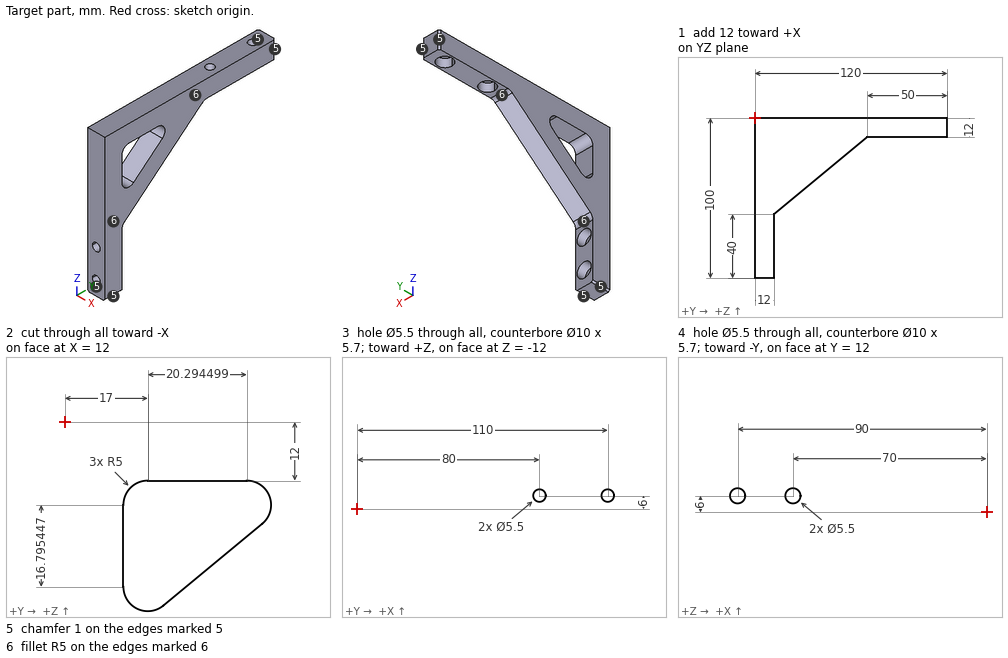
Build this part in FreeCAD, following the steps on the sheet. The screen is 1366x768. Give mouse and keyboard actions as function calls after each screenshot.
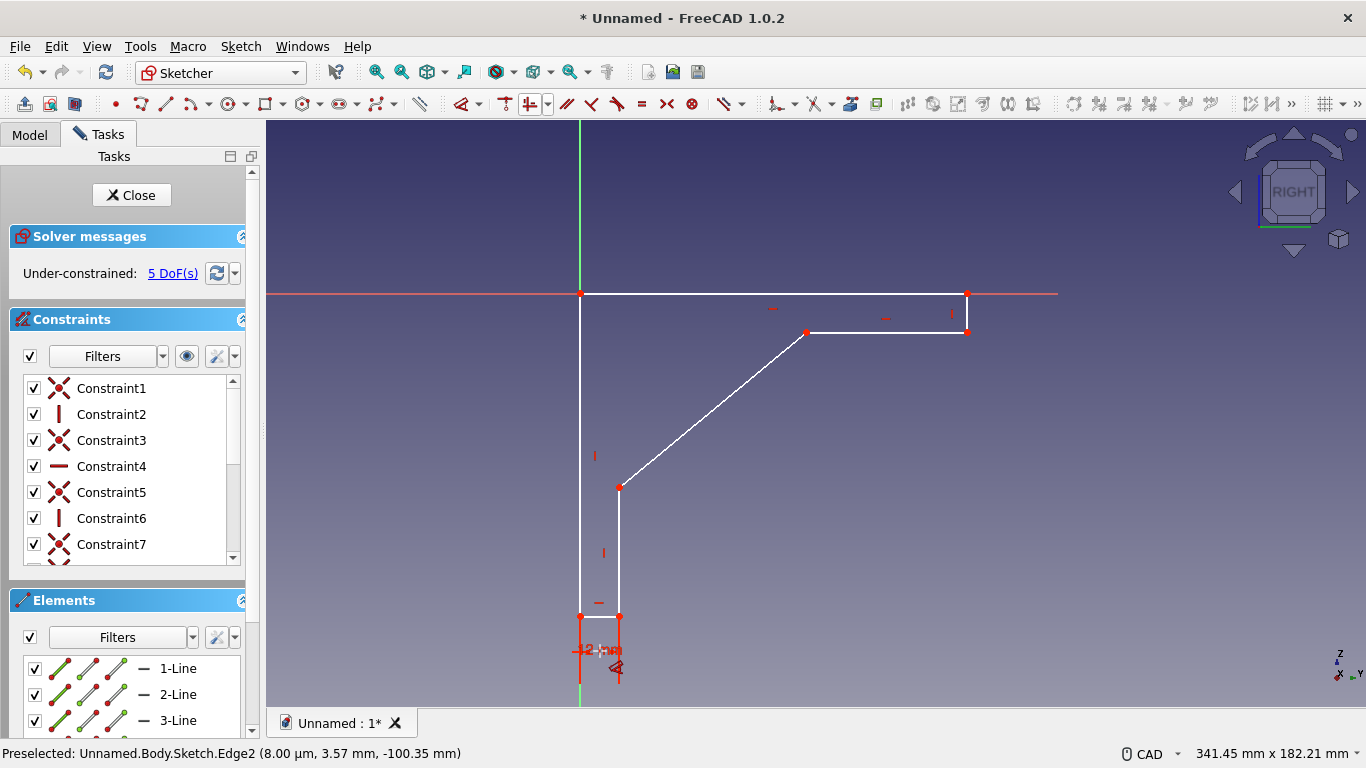
click(619, 578)
click(653, 553)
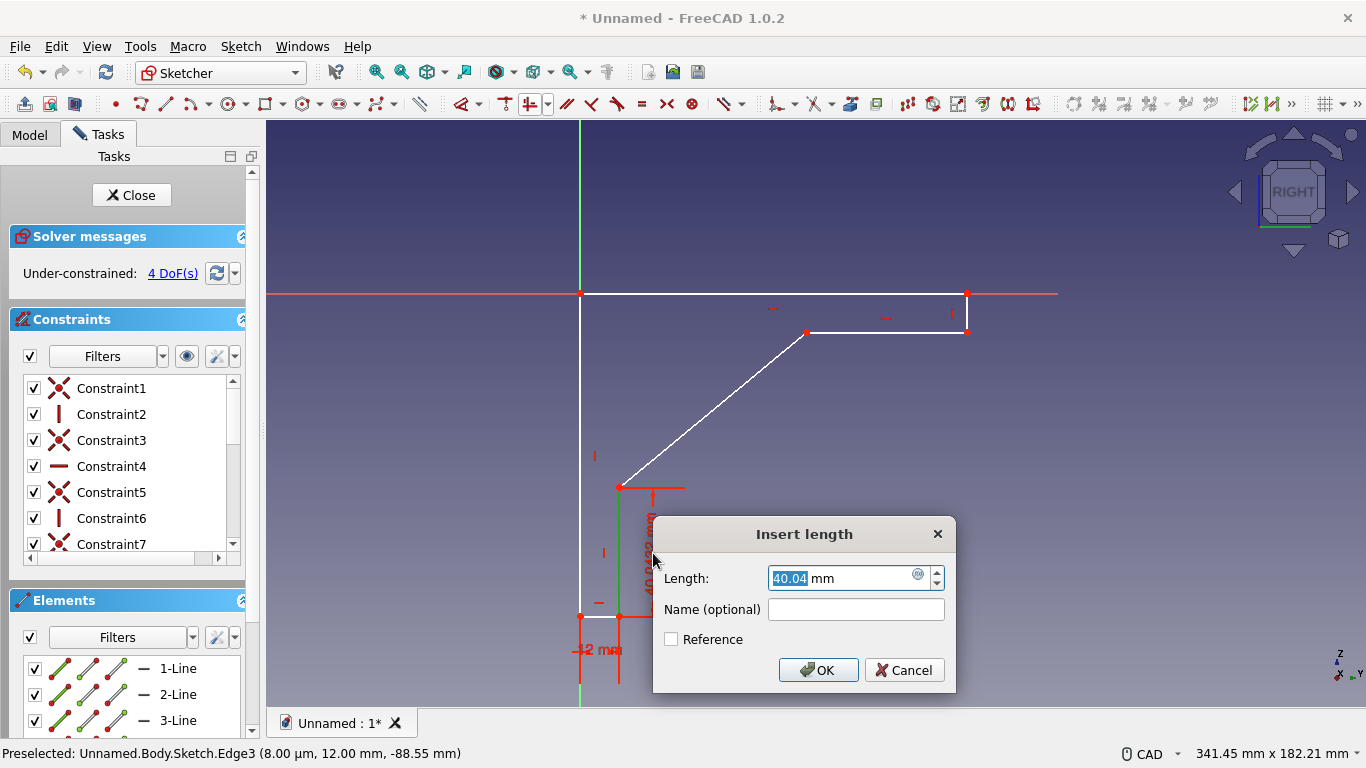
text(40)
key(Return)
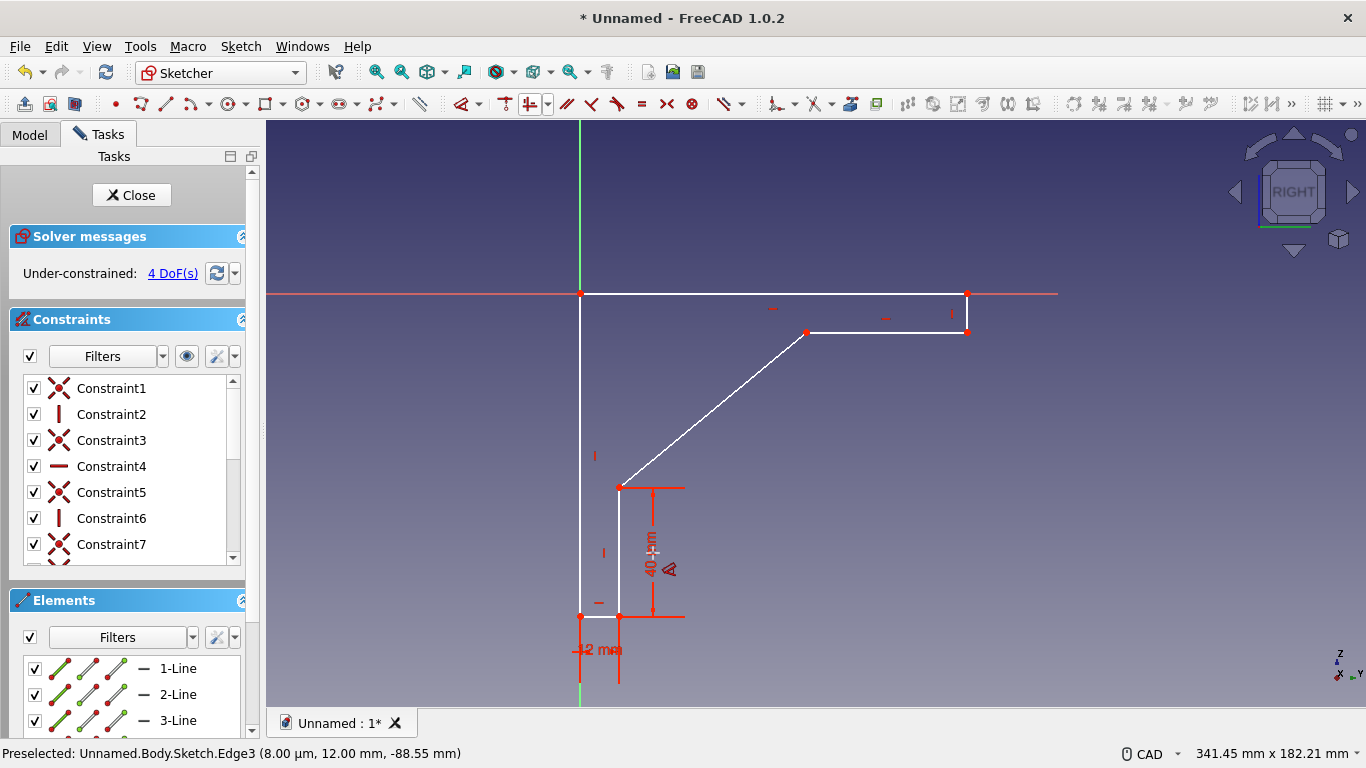
click(854, 333)
click(886, 367)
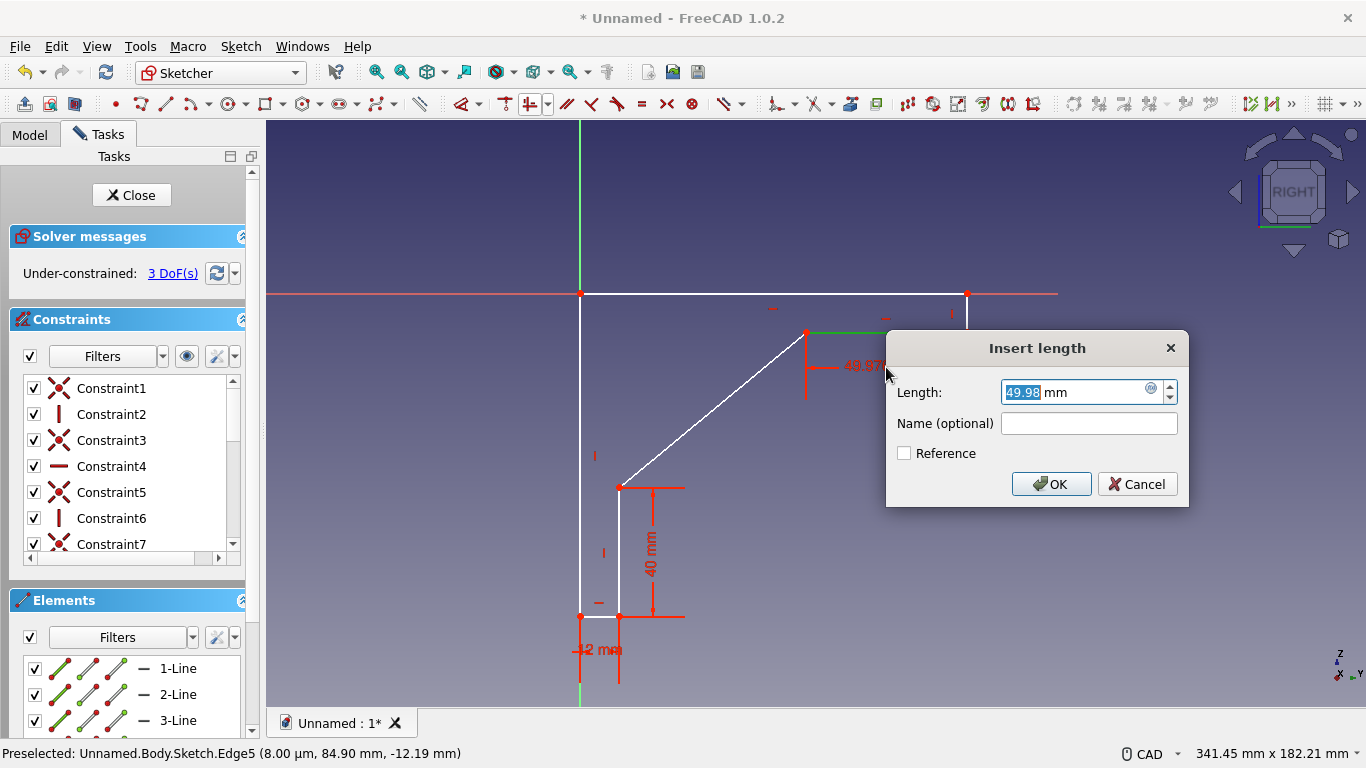
text(50)
key(Return)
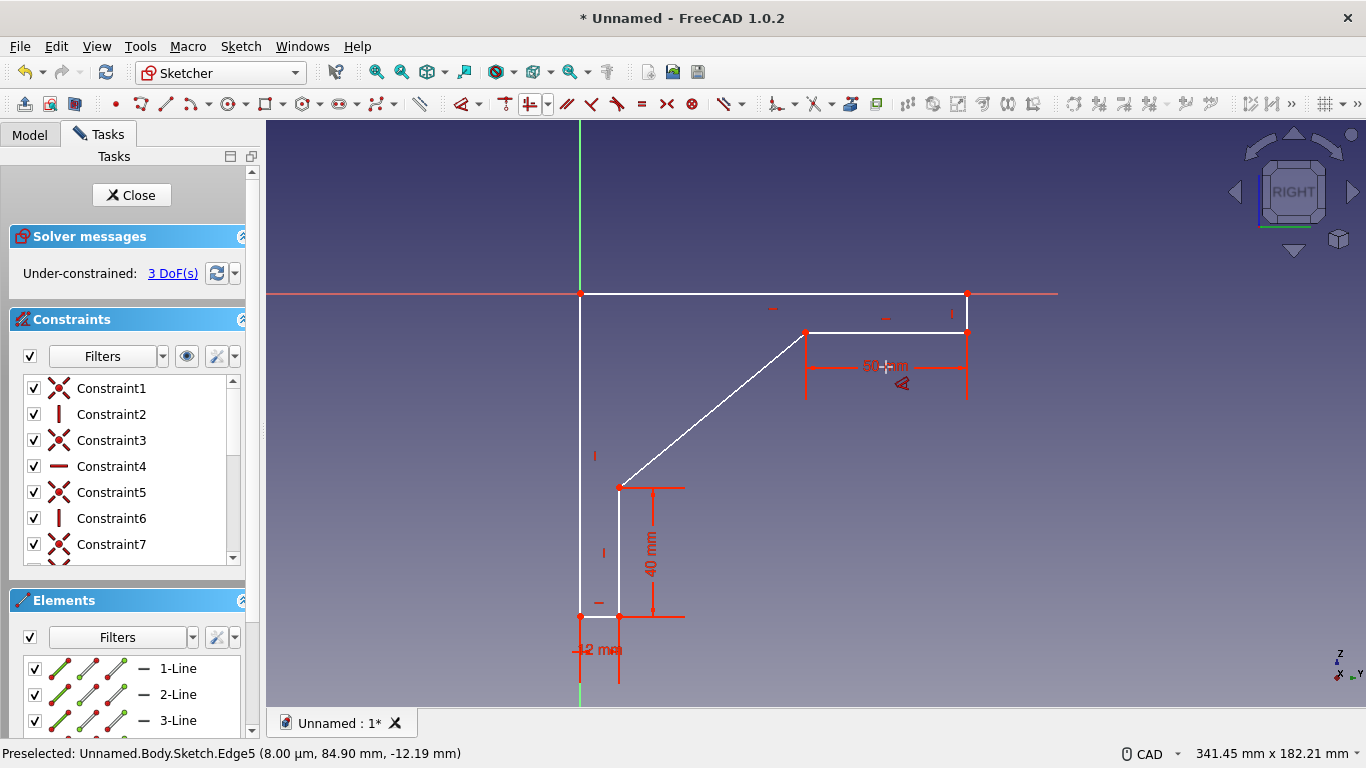
click(967, 321)
click(1001, 313)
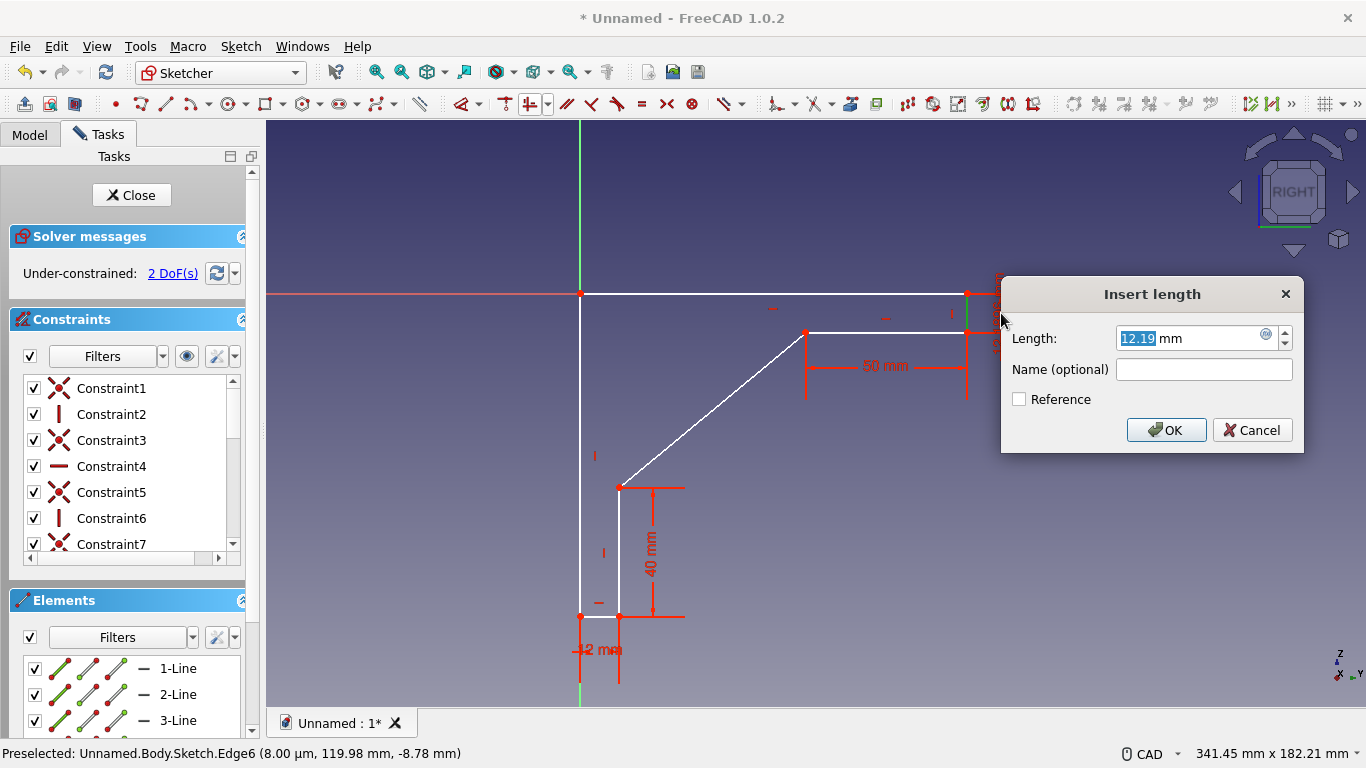
text(12)
key(Return)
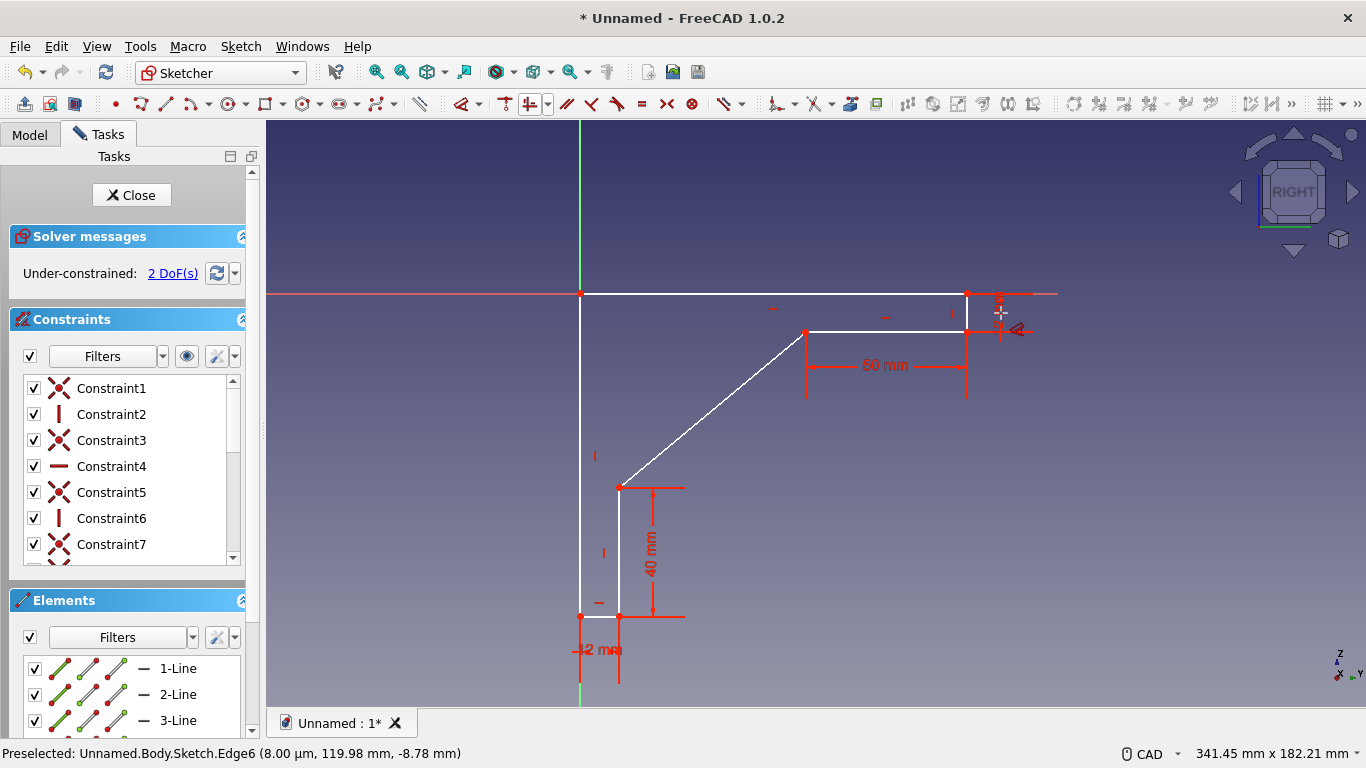
click(580, 391)
click(546, 455)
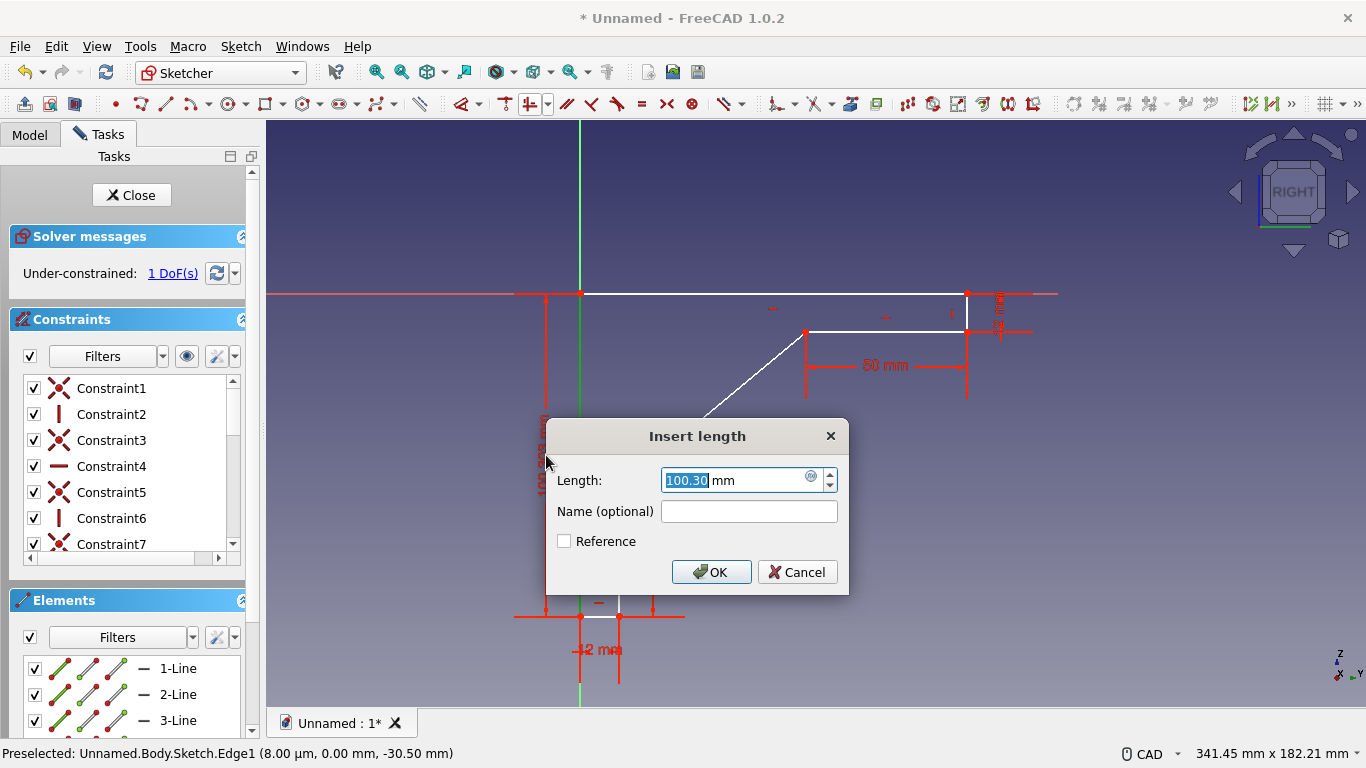
text(100)
key(Return)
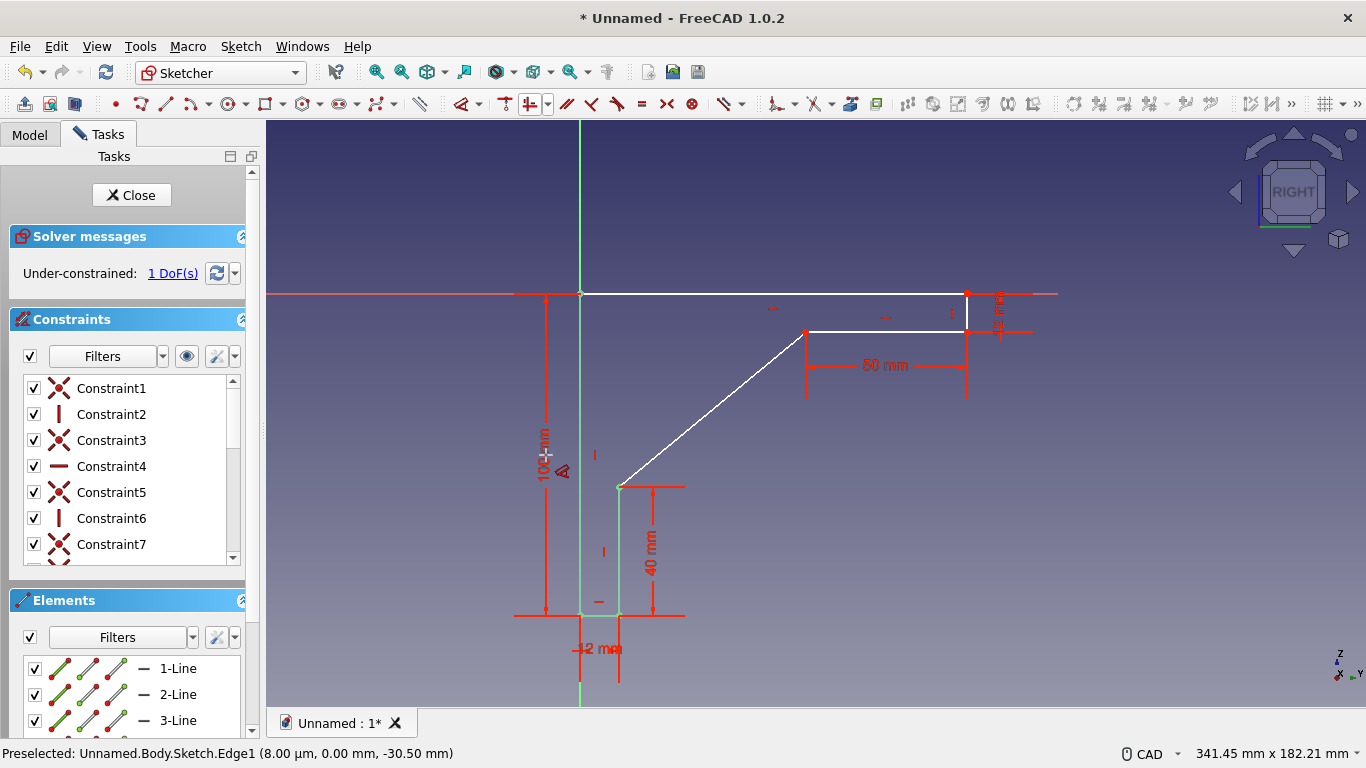
click(851, 294)
click(774, 260)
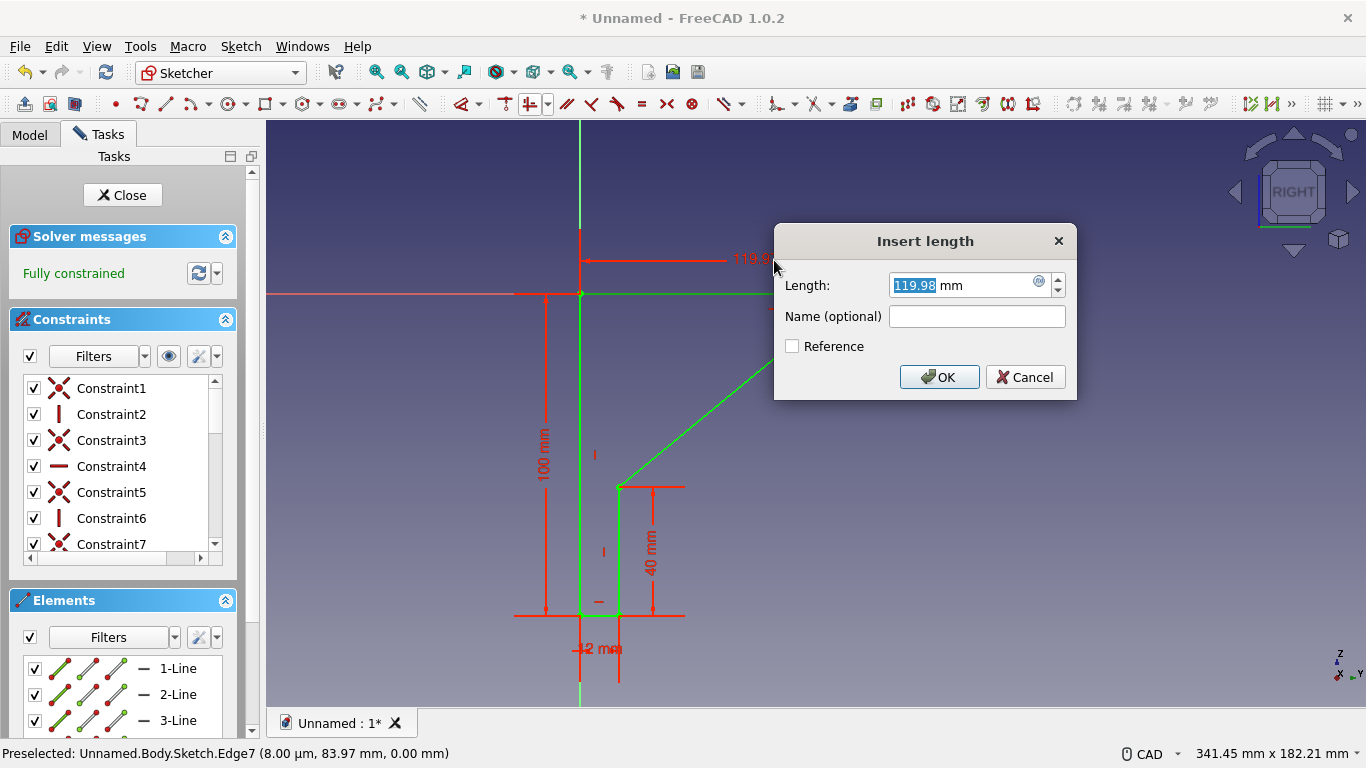
text(120)
key(Return)
key(Escape)